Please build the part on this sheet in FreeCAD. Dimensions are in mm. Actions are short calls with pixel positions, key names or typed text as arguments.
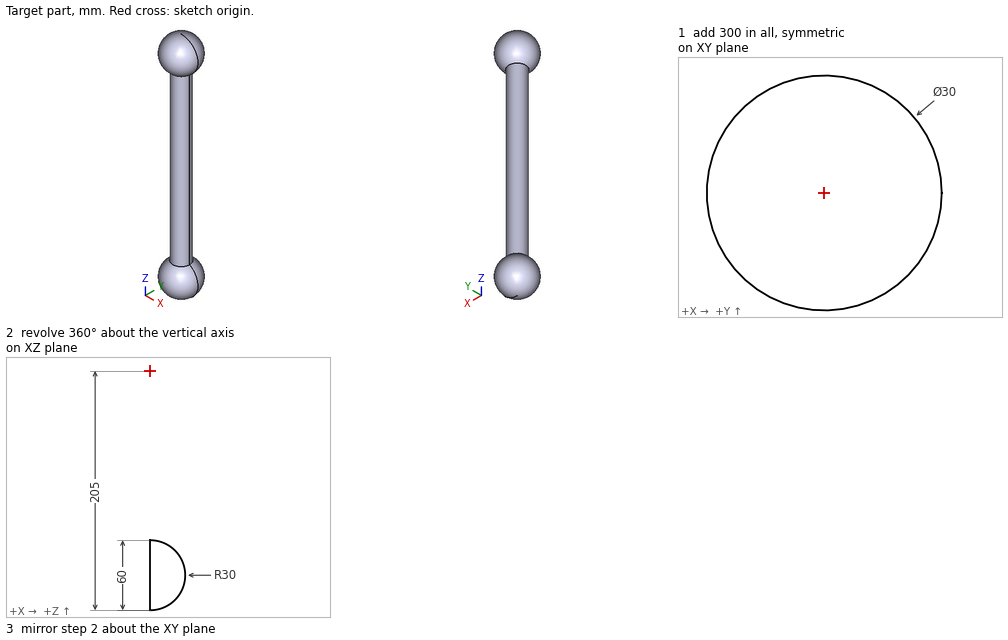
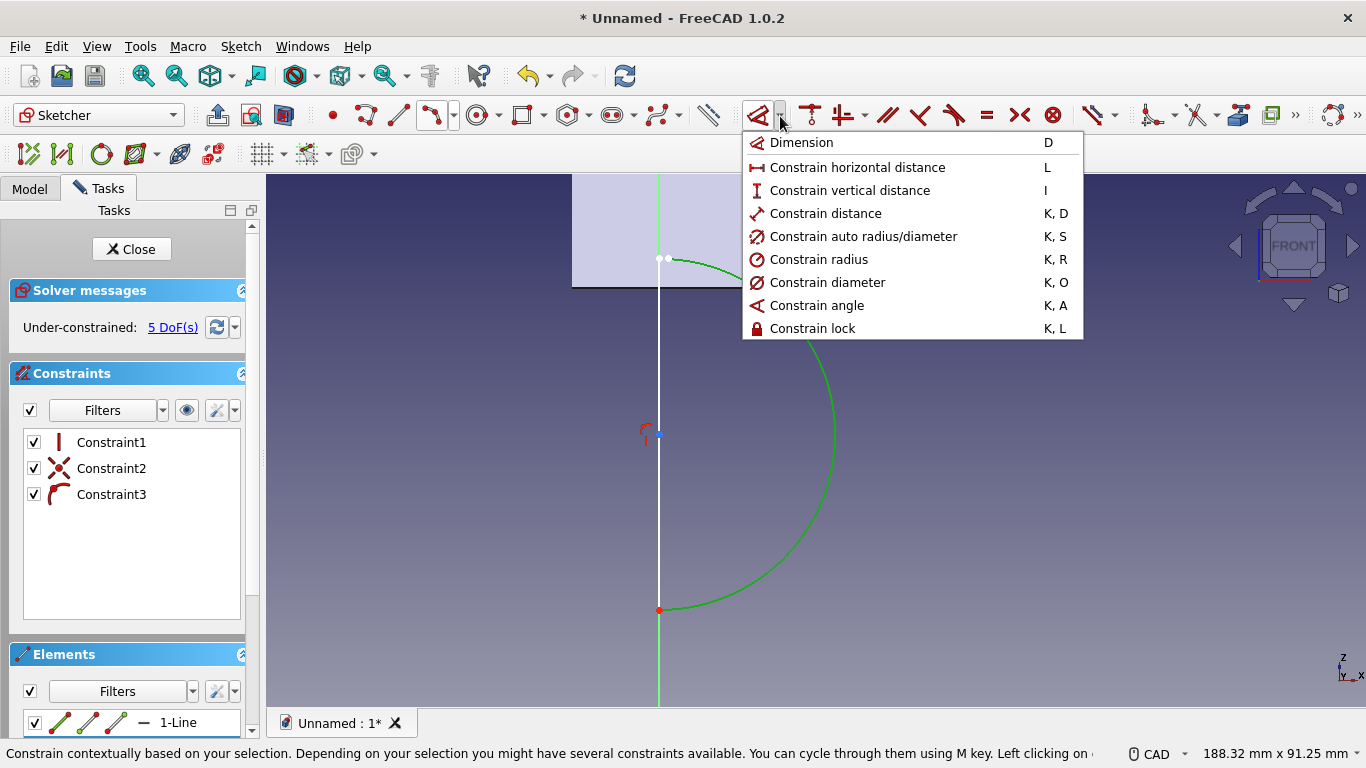
click(913, 260)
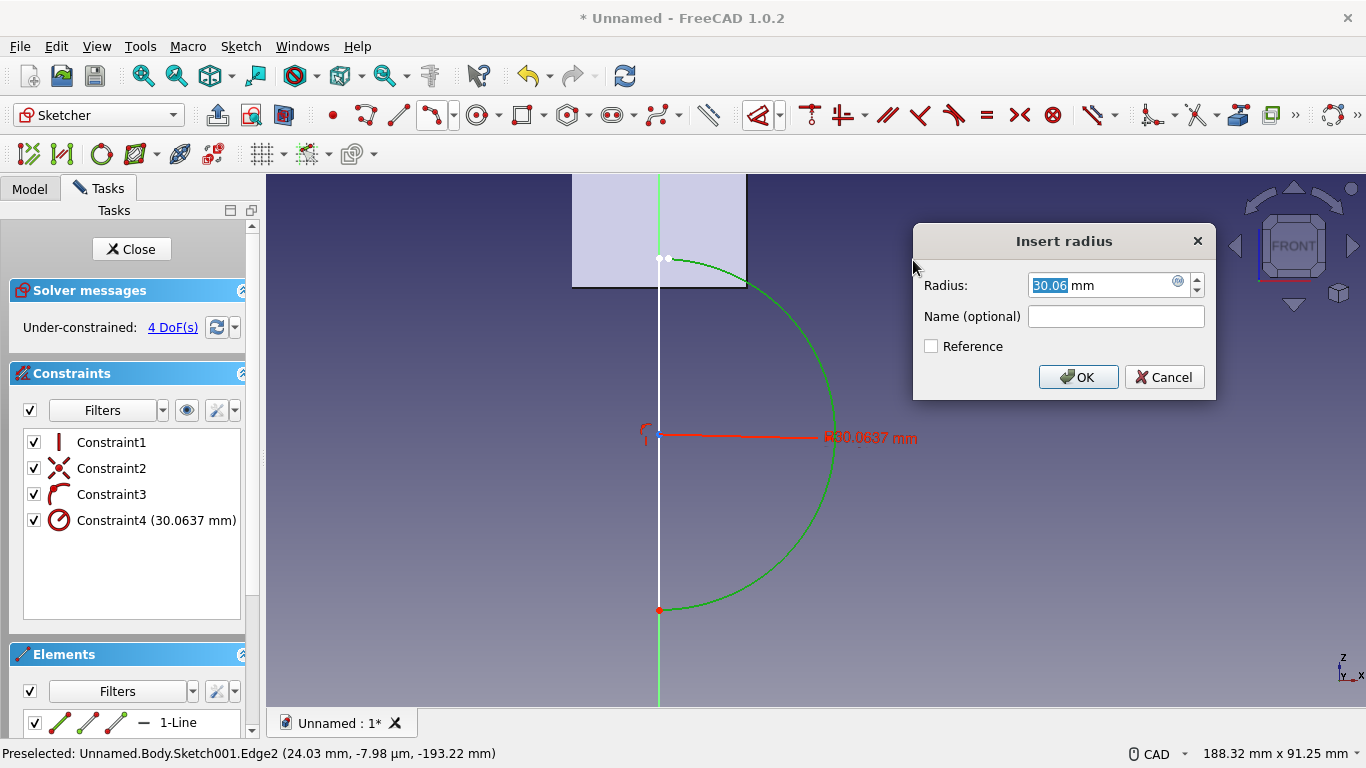
text(30)
key(Return)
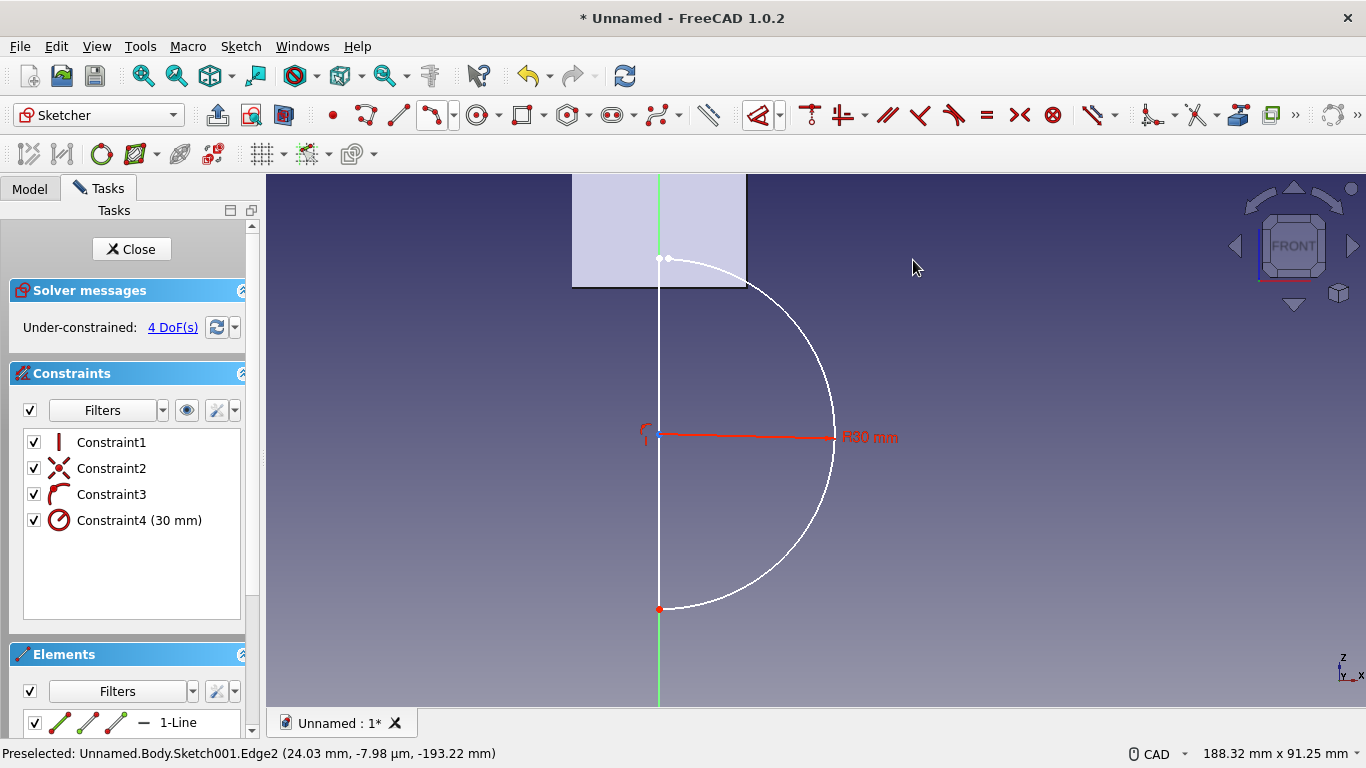
click(659, 609)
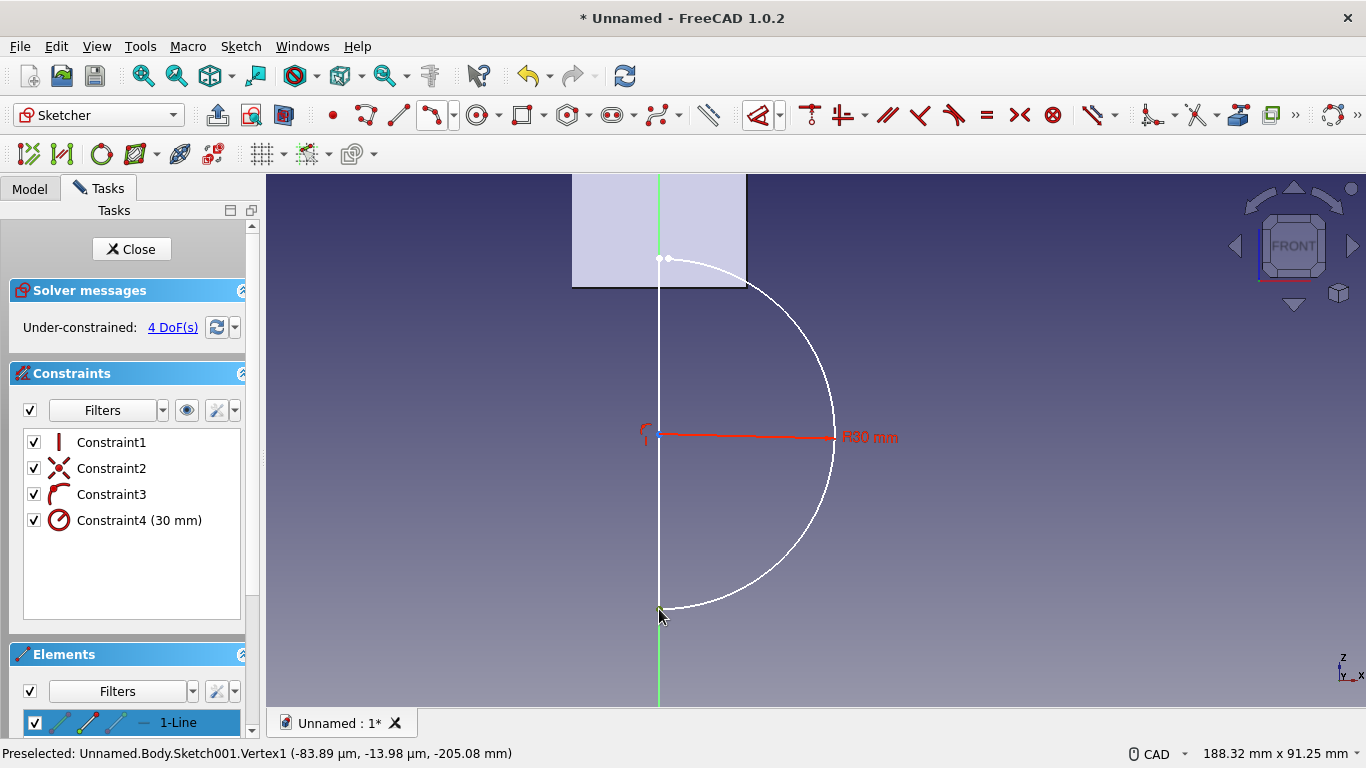
click(659, 645)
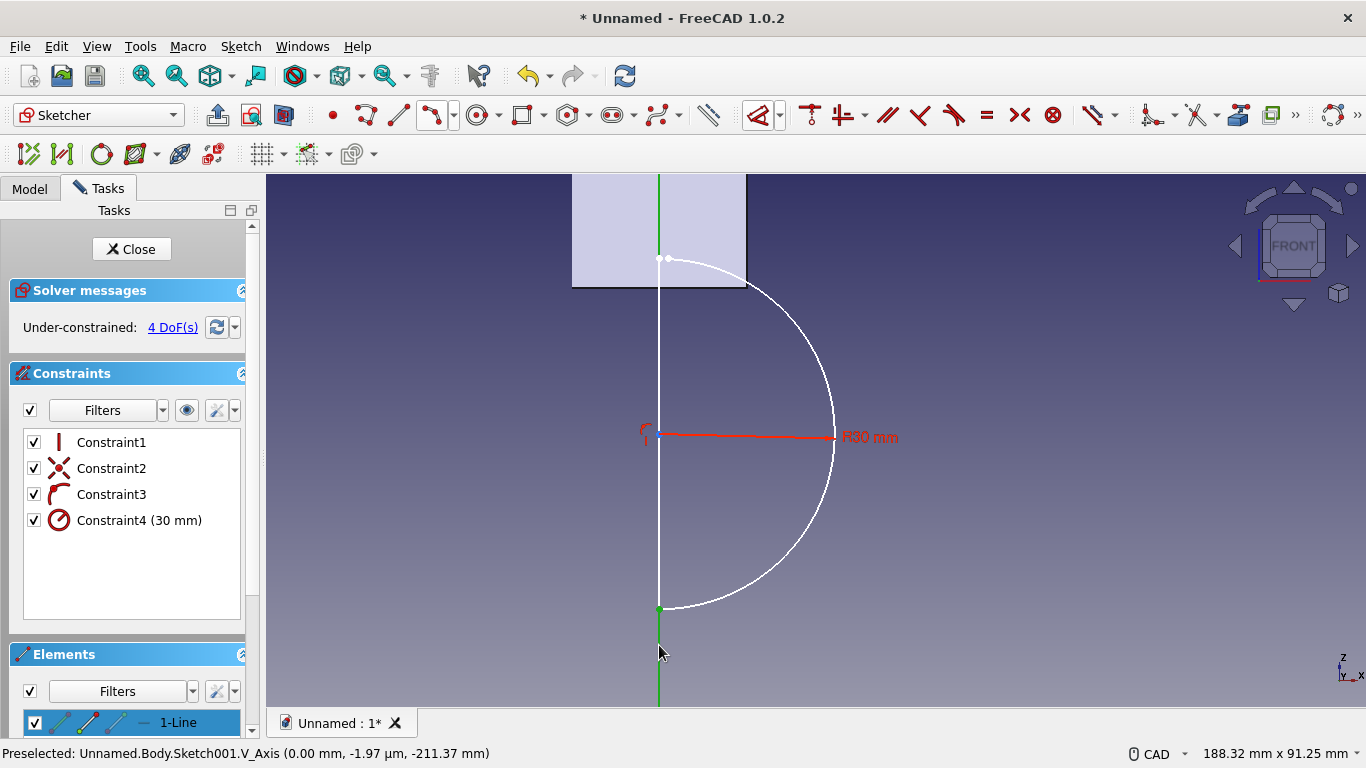
click(810, 116)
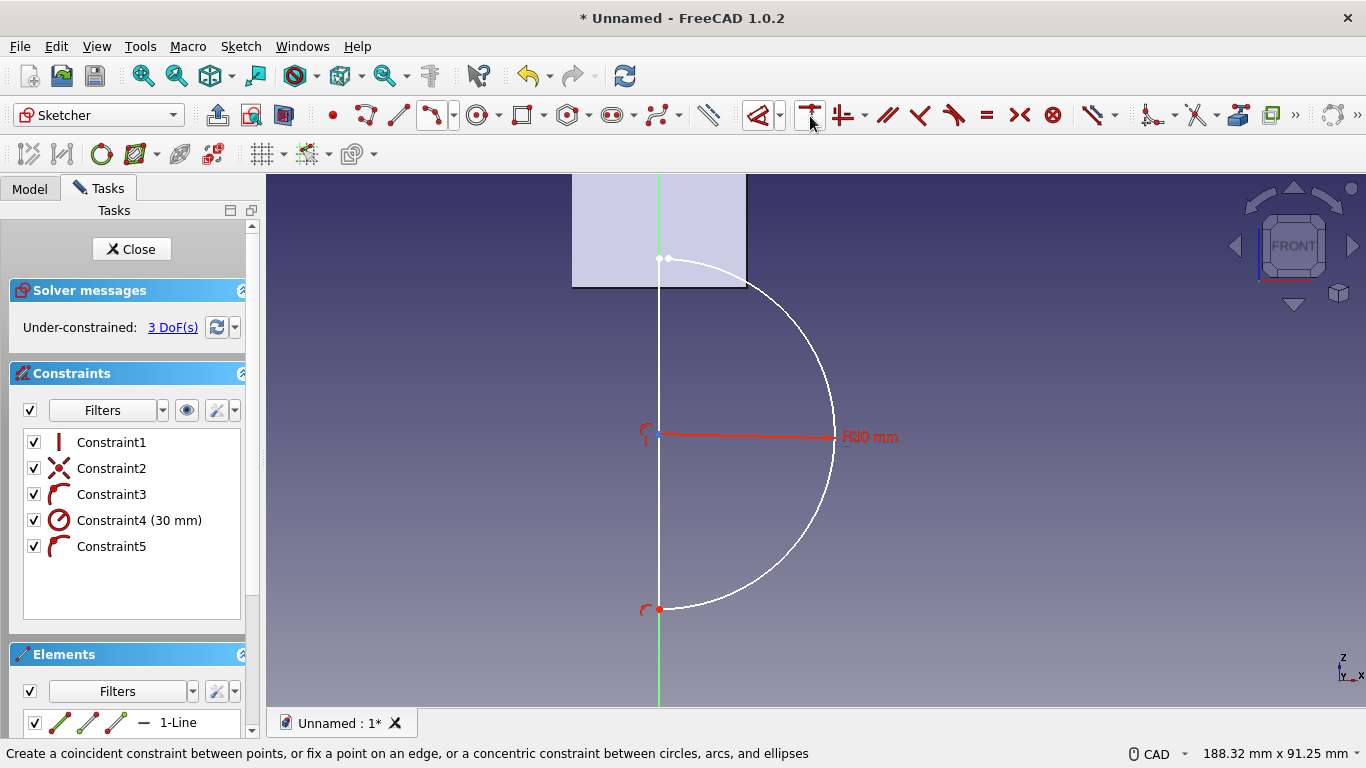
click(668, 259)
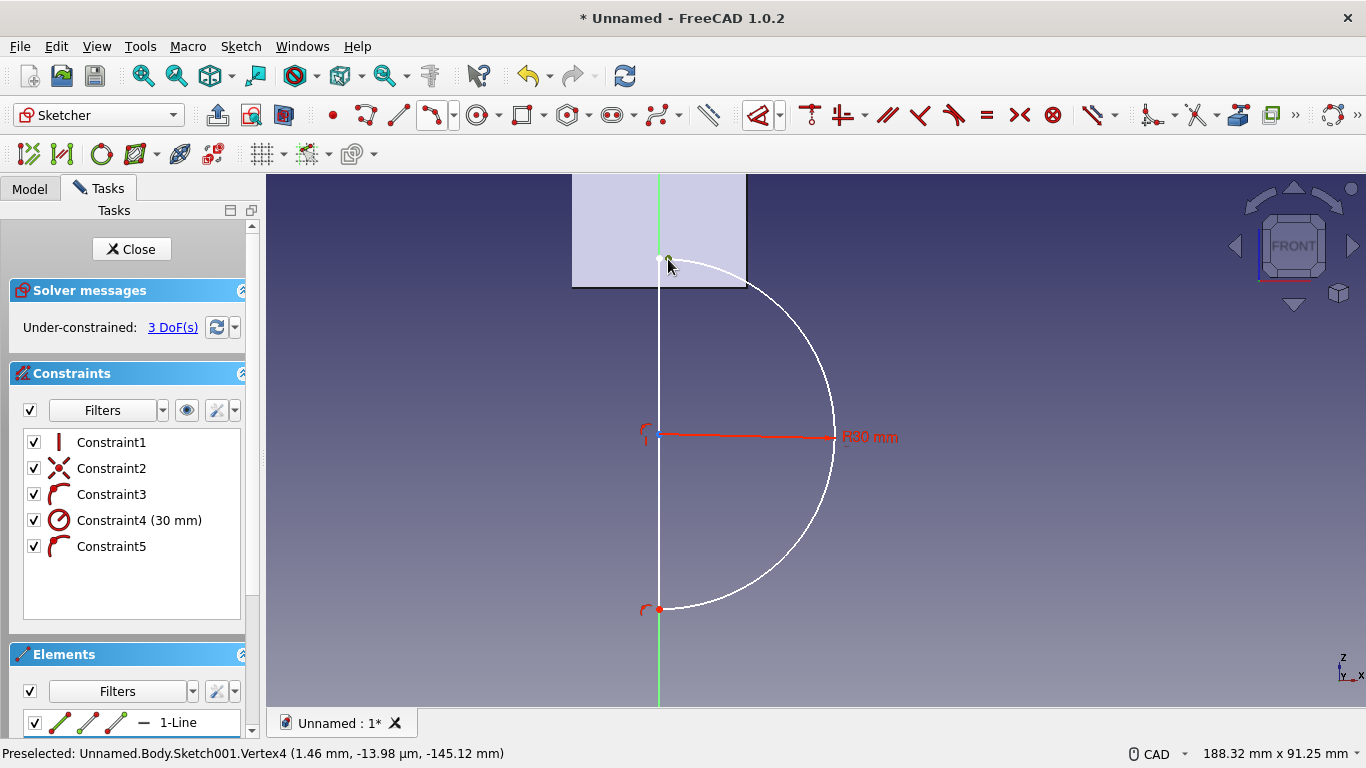
click(659, 645)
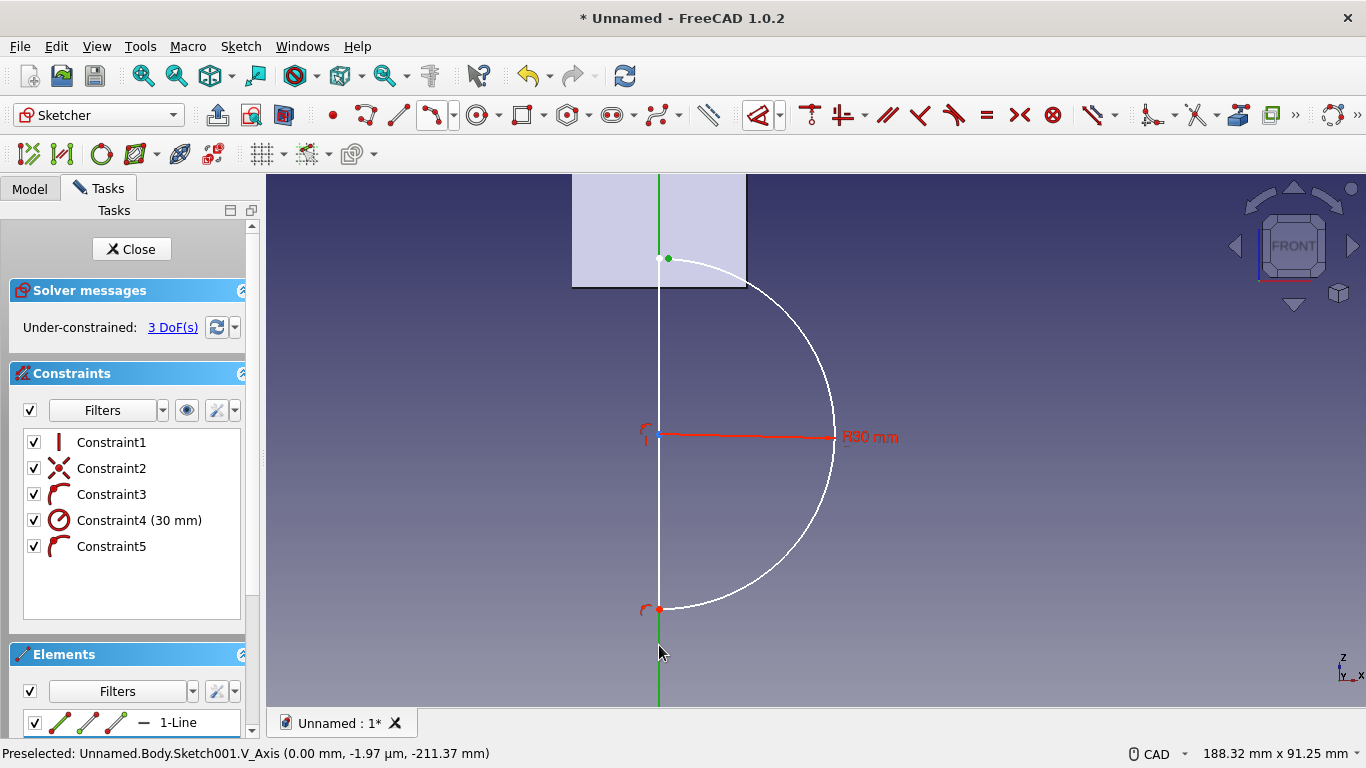
click(810, 116)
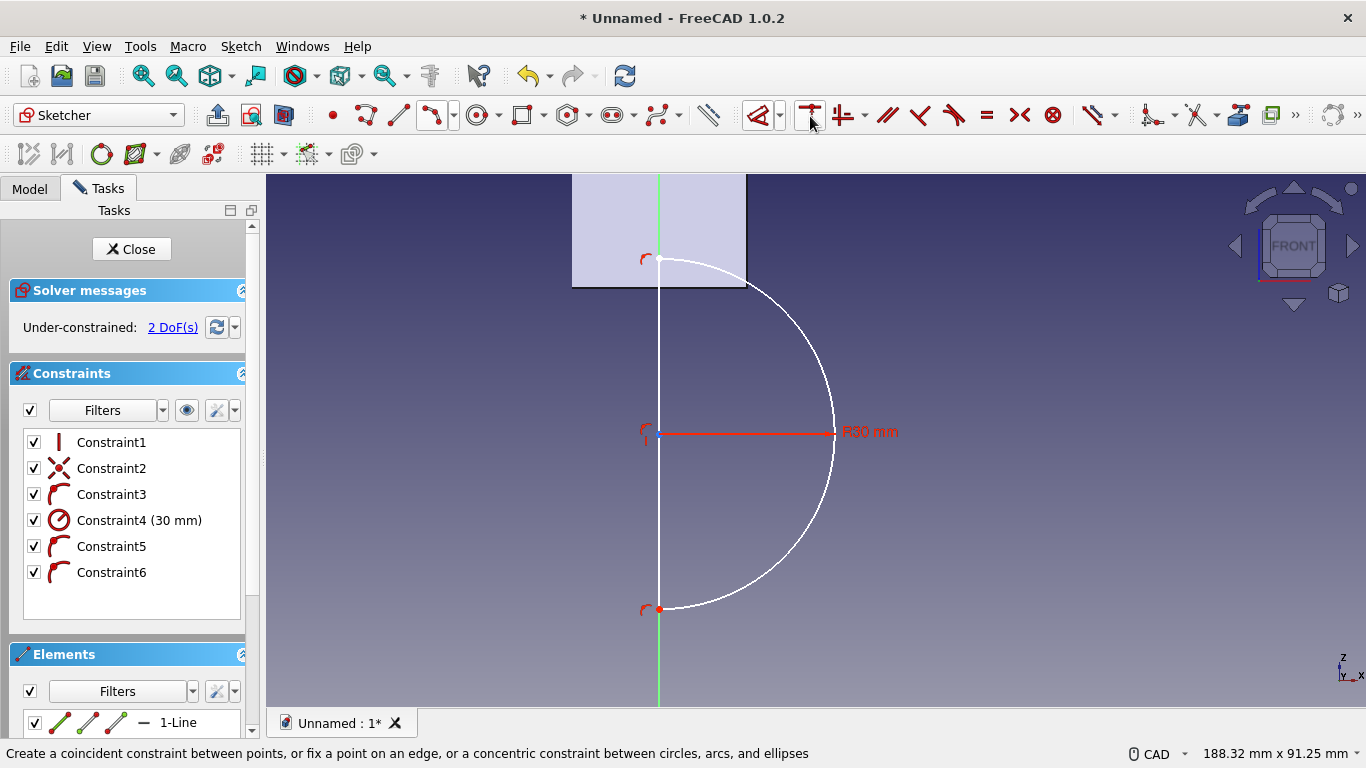
click(659, 504)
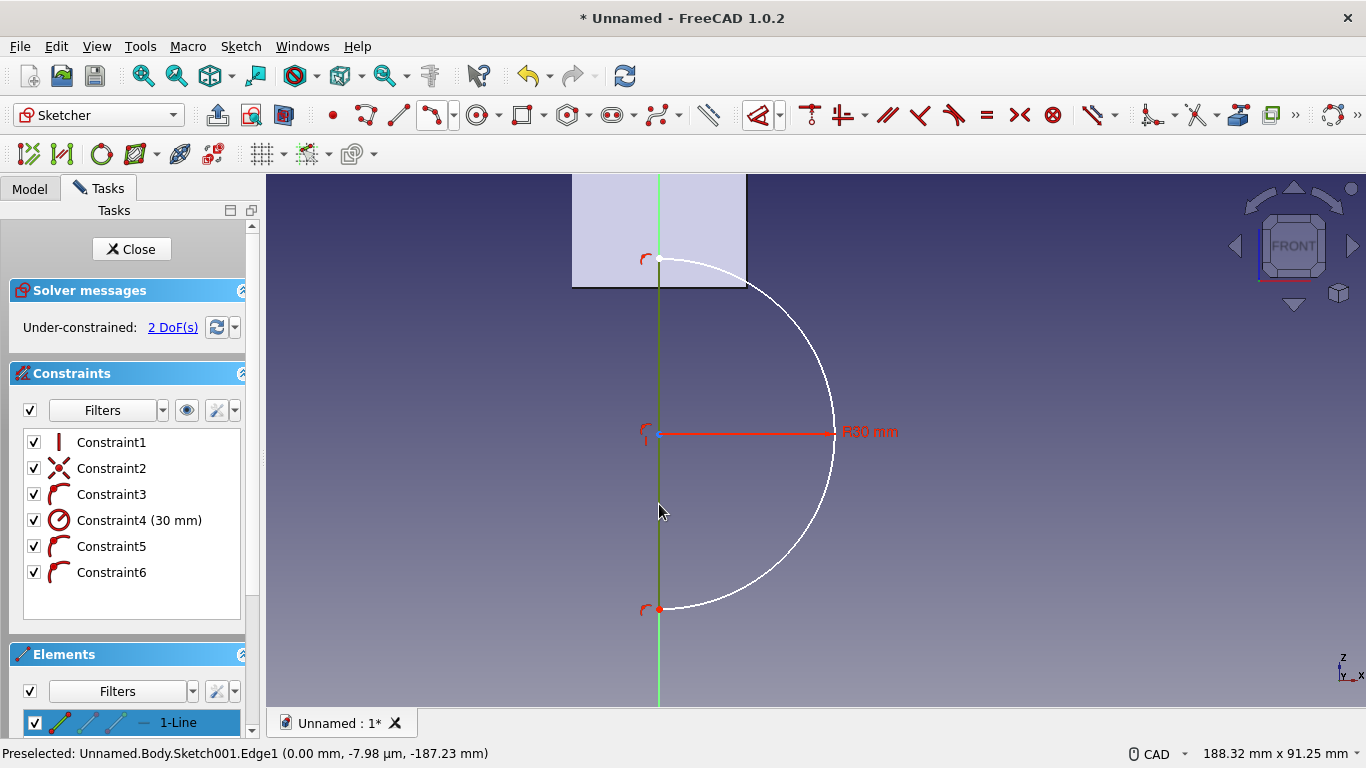
key(i)